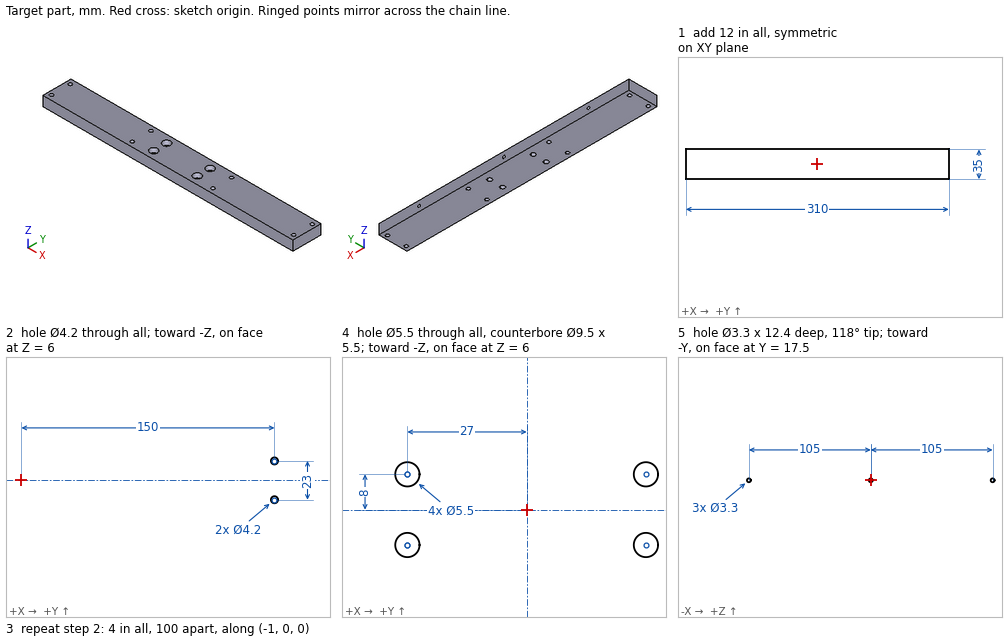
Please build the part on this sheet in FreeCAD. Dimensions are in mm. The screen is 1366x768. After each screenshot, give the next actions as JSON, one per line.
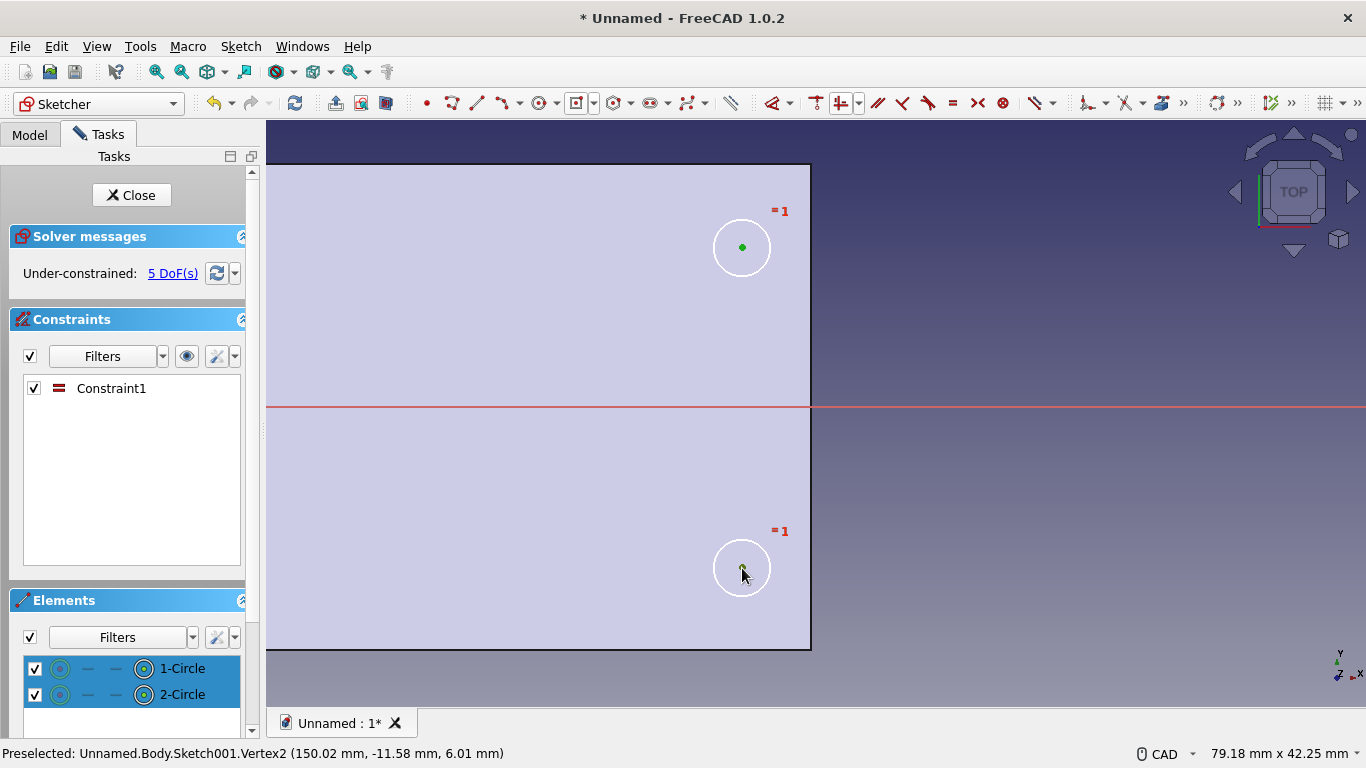
{"action": "left_click", "coordinate": [359, 407]}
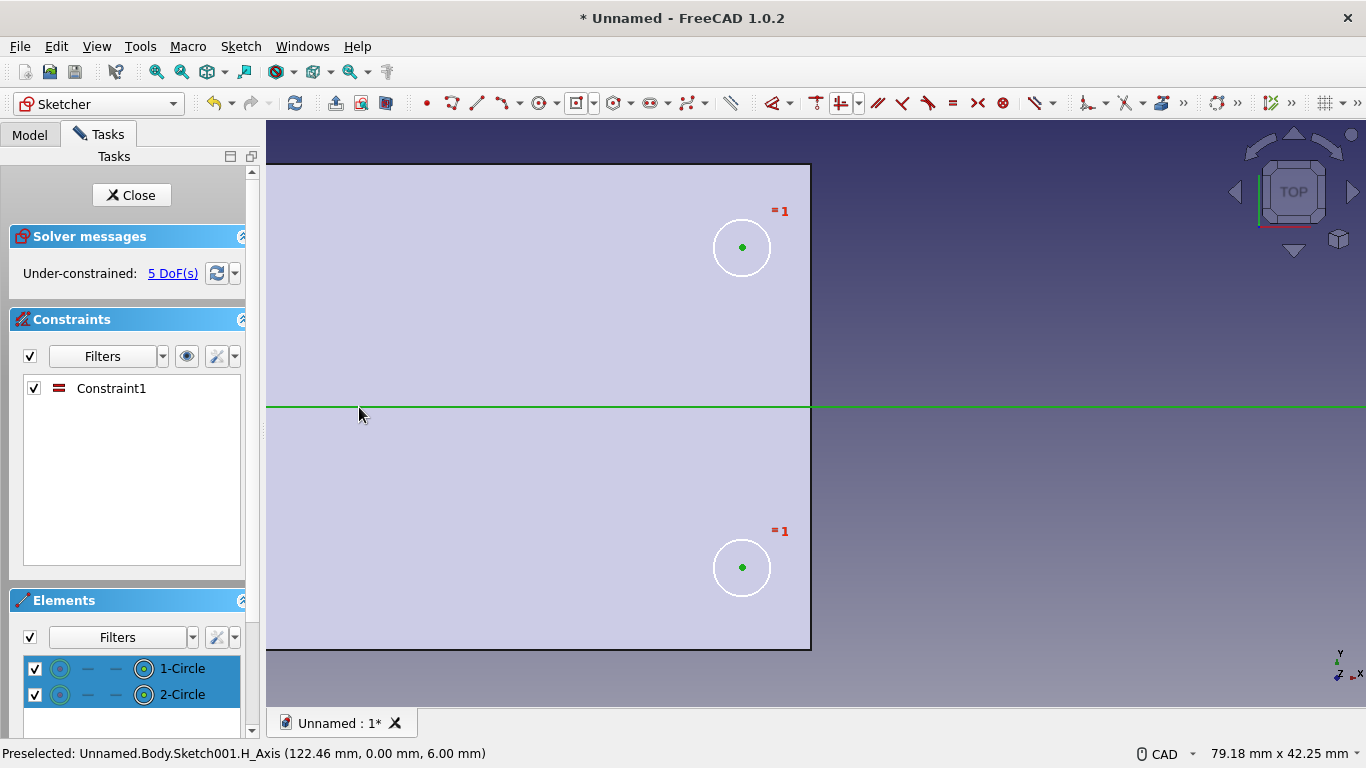
{"action": "left_click", "coordinate": [978, 104]}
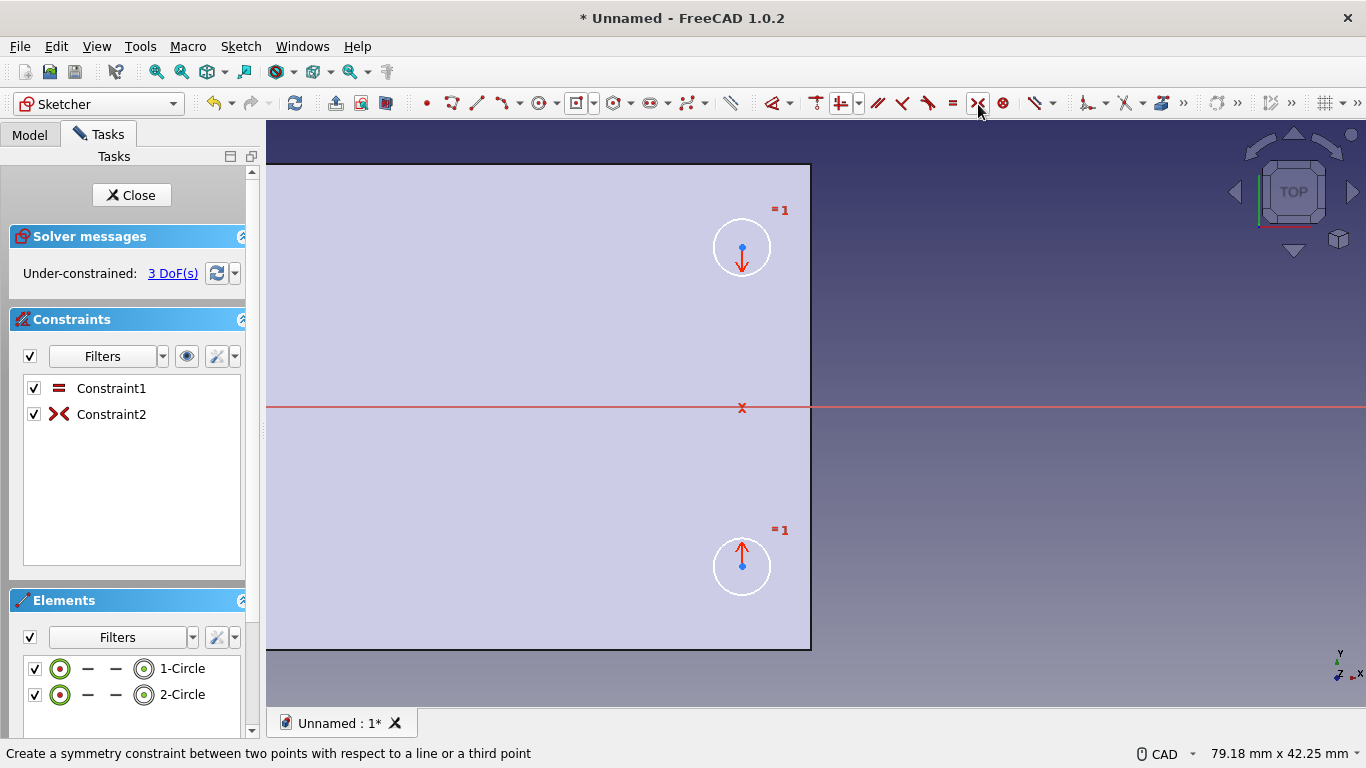
{"action": "key", "text": "d"}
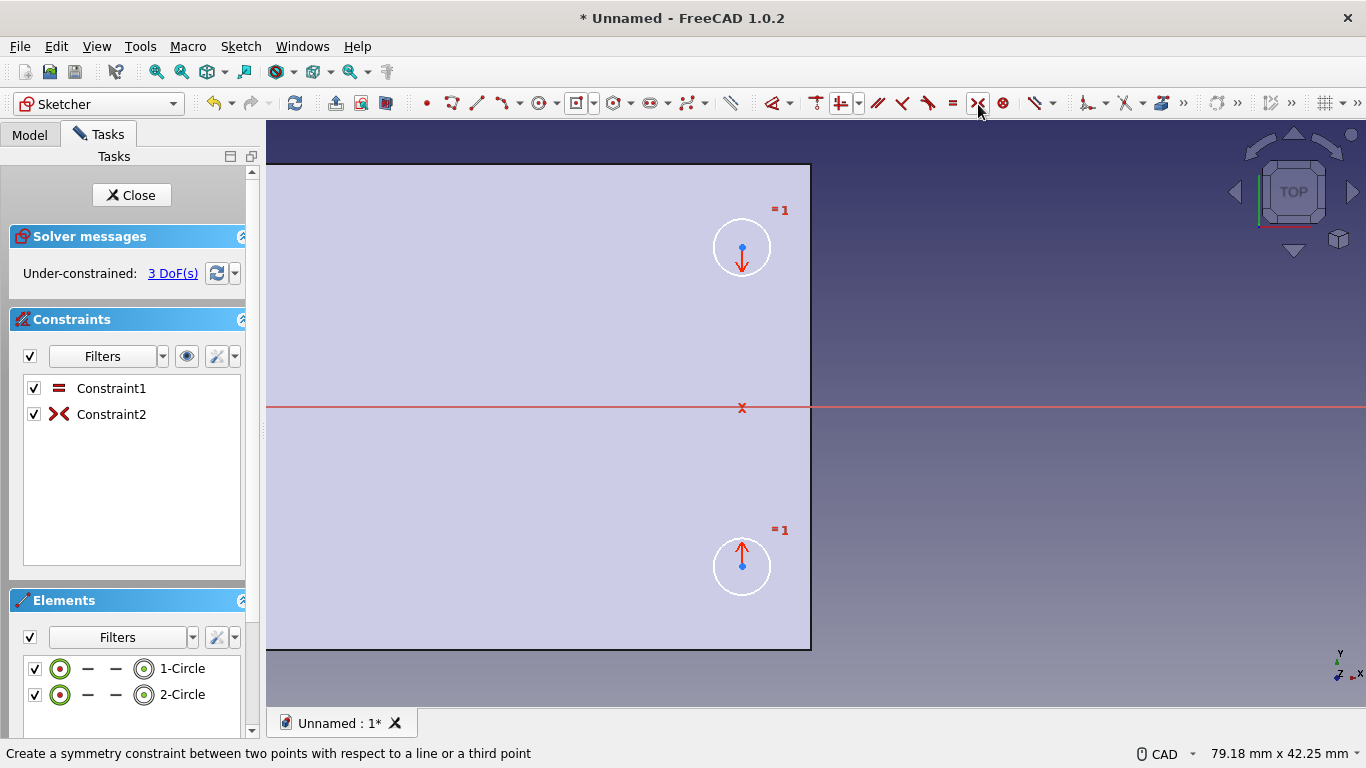
{"action": "left_click", "coordinate": [762, 227]}
{"action": "left_click", "coordinate": [784, 204]}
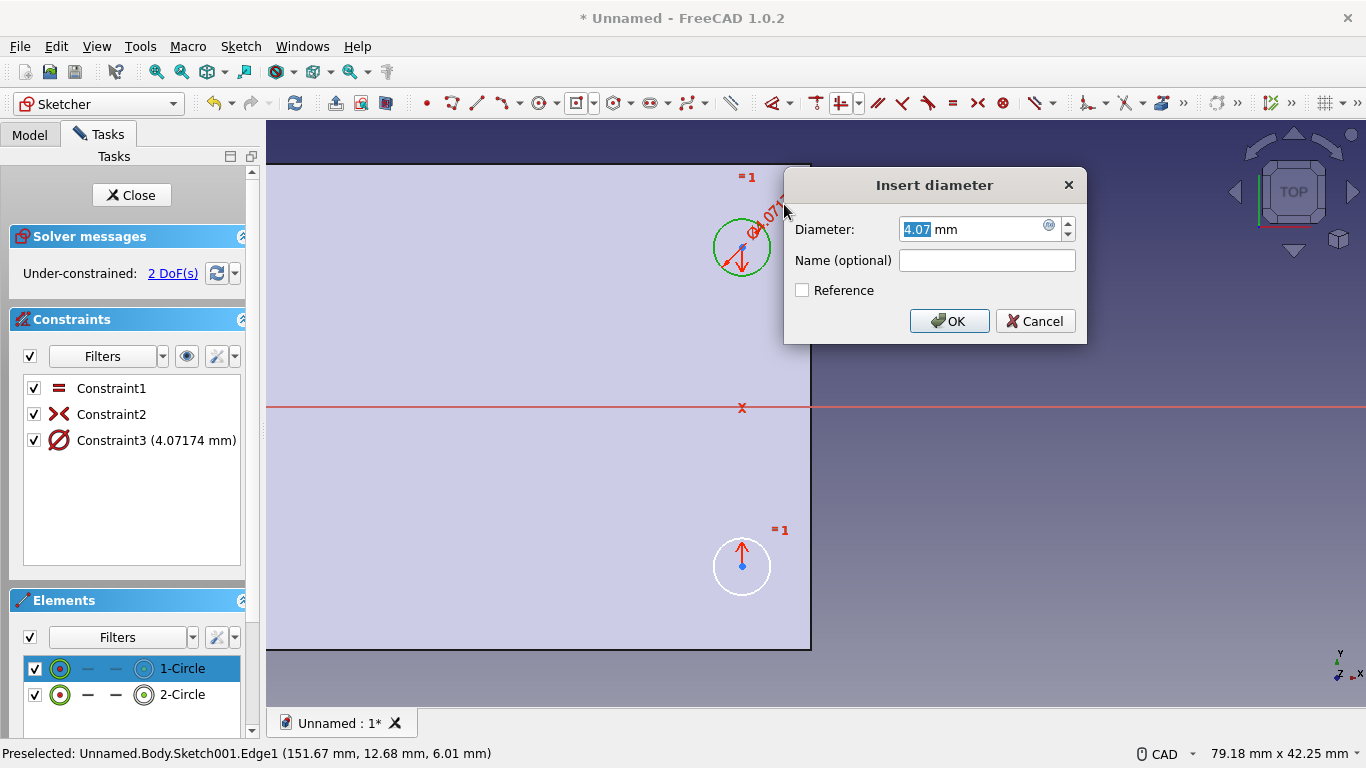
{"action": "type", "text": "4.2"}
{"action": "key", "text": "Return"}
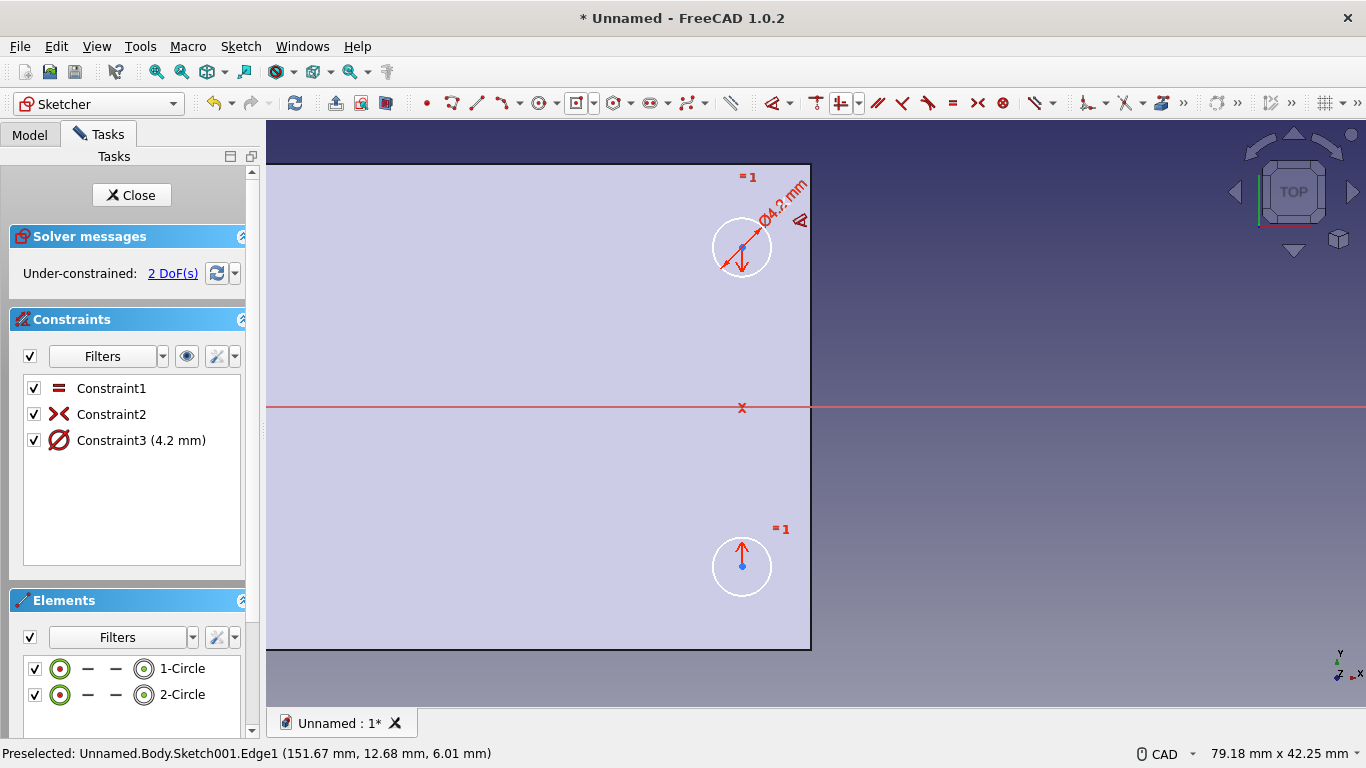
{"action": "left_click", "coordinate": [742, 247]}
{"action": "left_click", "coordinate": [518, 213]}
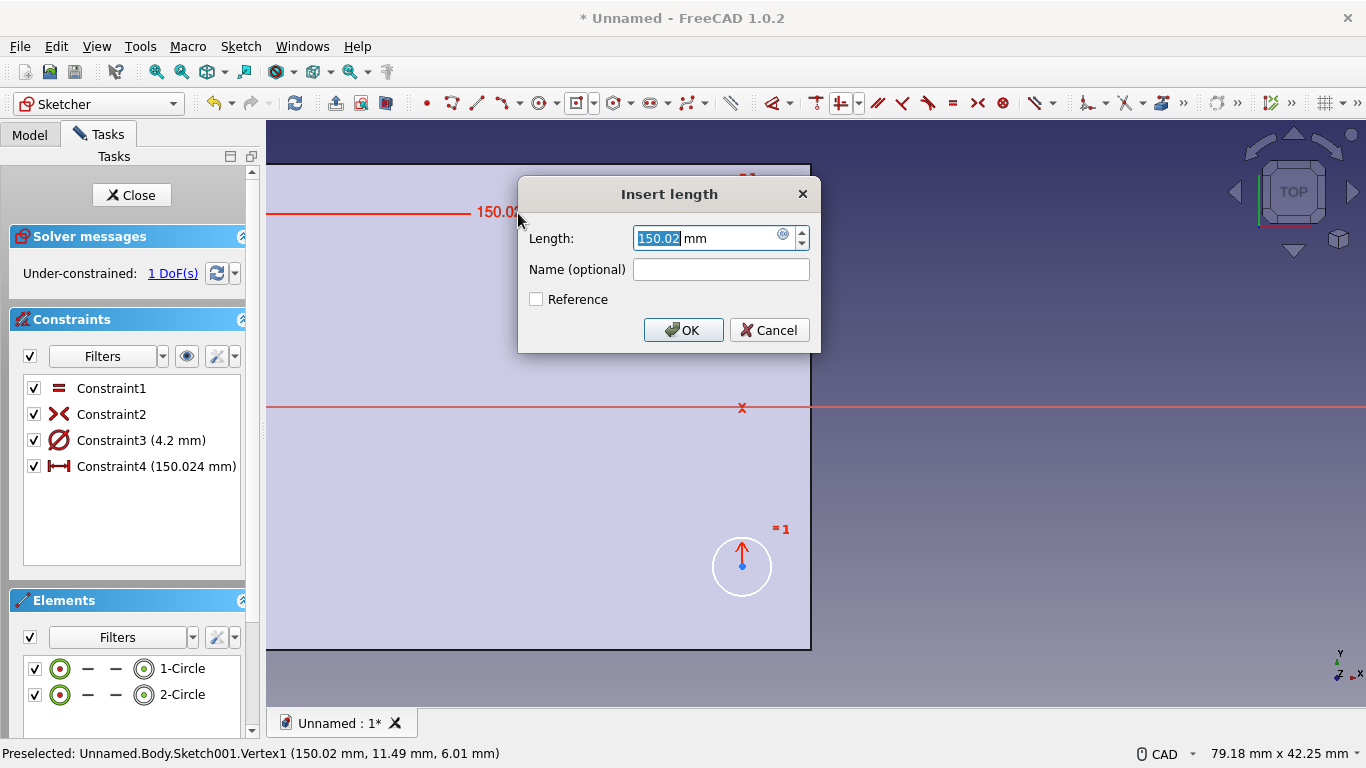
{"action": "type", "text": "150"}
{"action": "key", "text": "Return"}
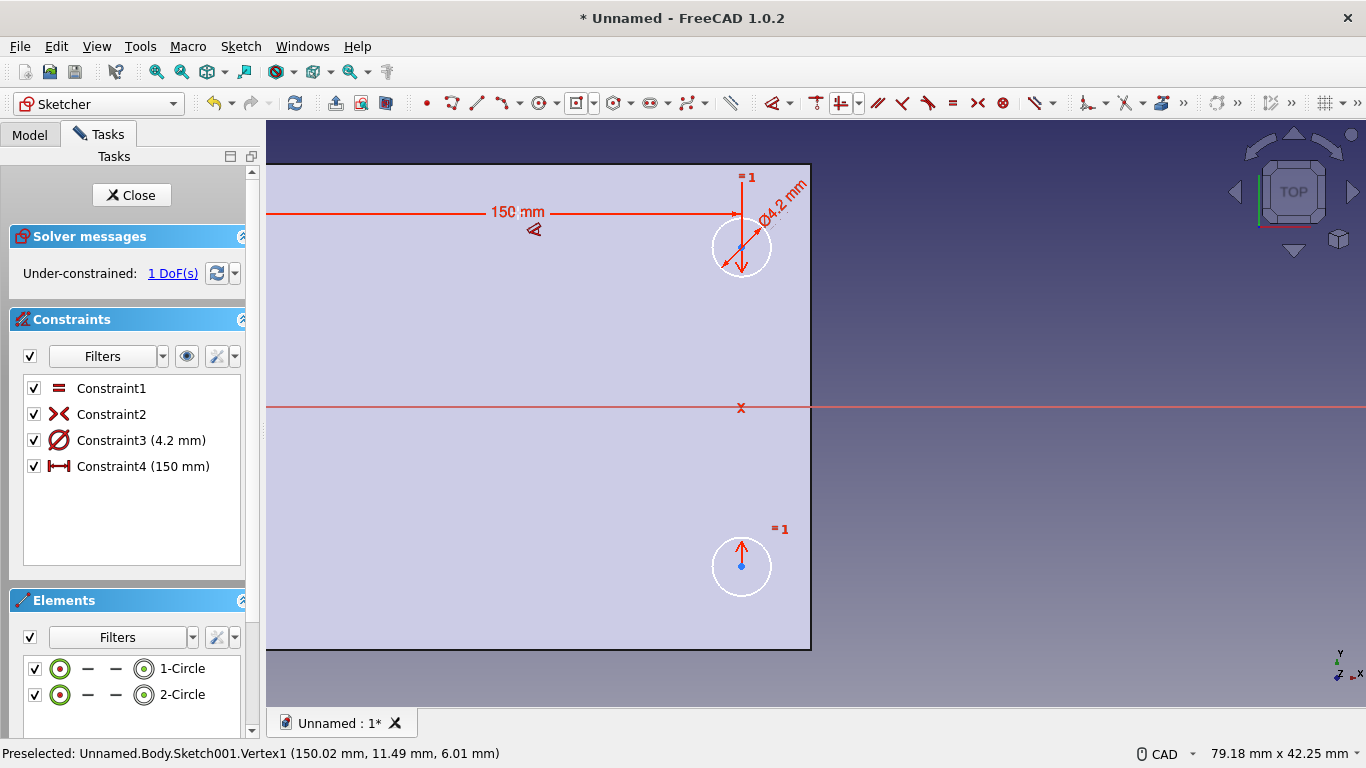
{"action": "left_click", "coordinate": [742, 247]}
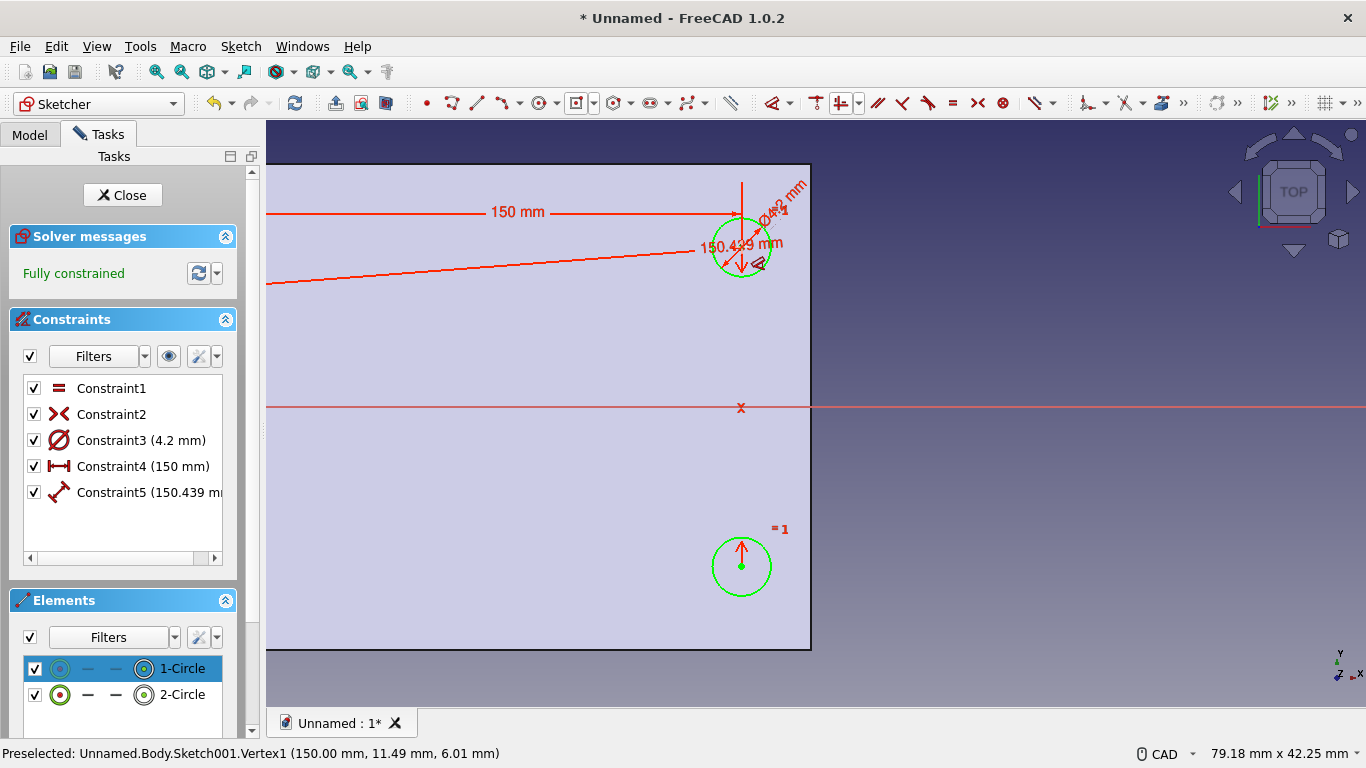
{"action": "left_click", "coordinate": [742, 567]}
{"action": "left_click", "coordinate": [776, 334]}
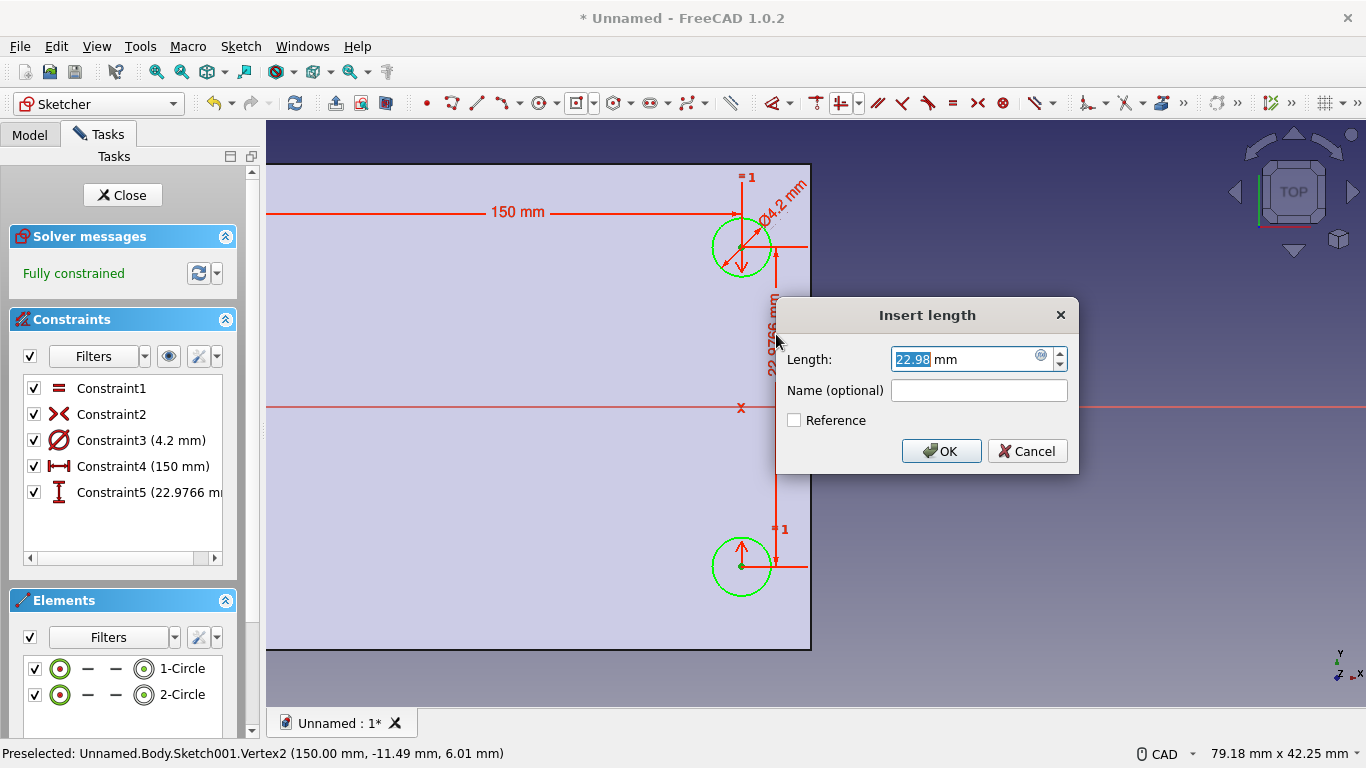
{"action": "type", "text": "23"}
{"action": "key", "text": "Return"}
{"action": "key", "text": "Escape"}